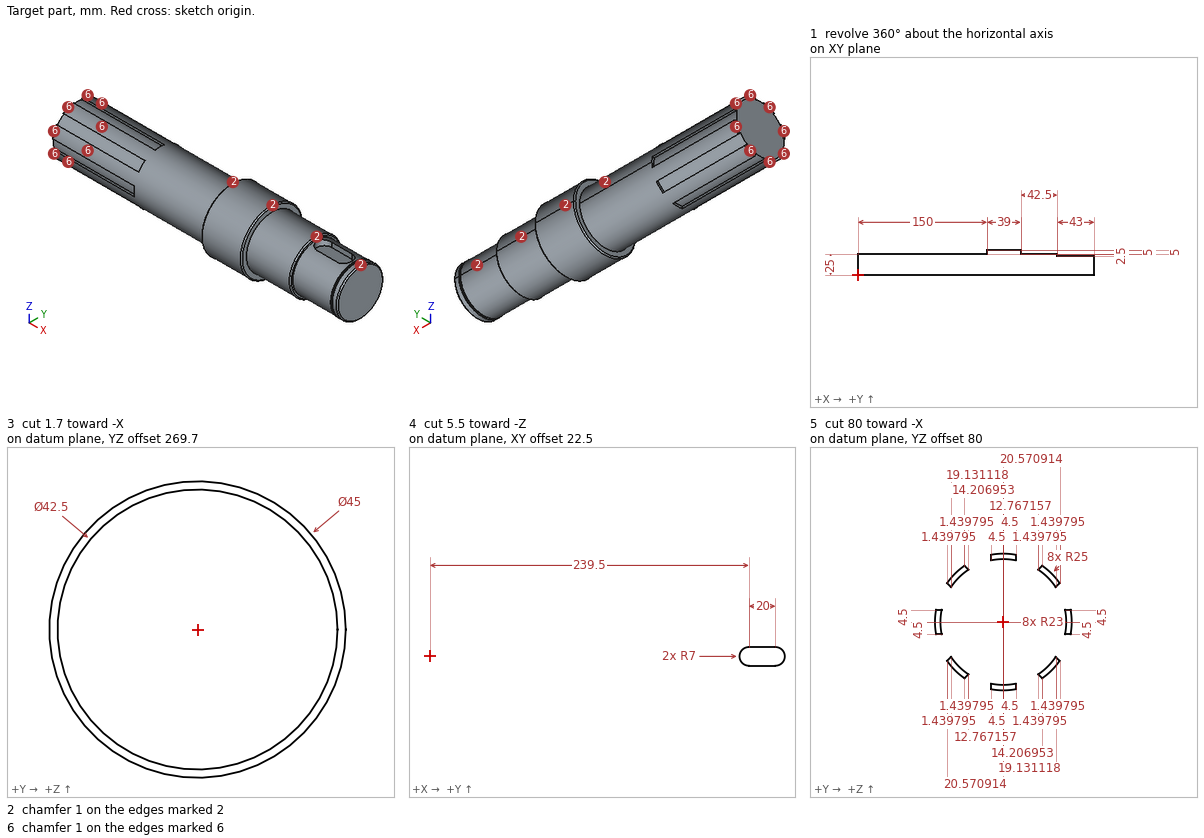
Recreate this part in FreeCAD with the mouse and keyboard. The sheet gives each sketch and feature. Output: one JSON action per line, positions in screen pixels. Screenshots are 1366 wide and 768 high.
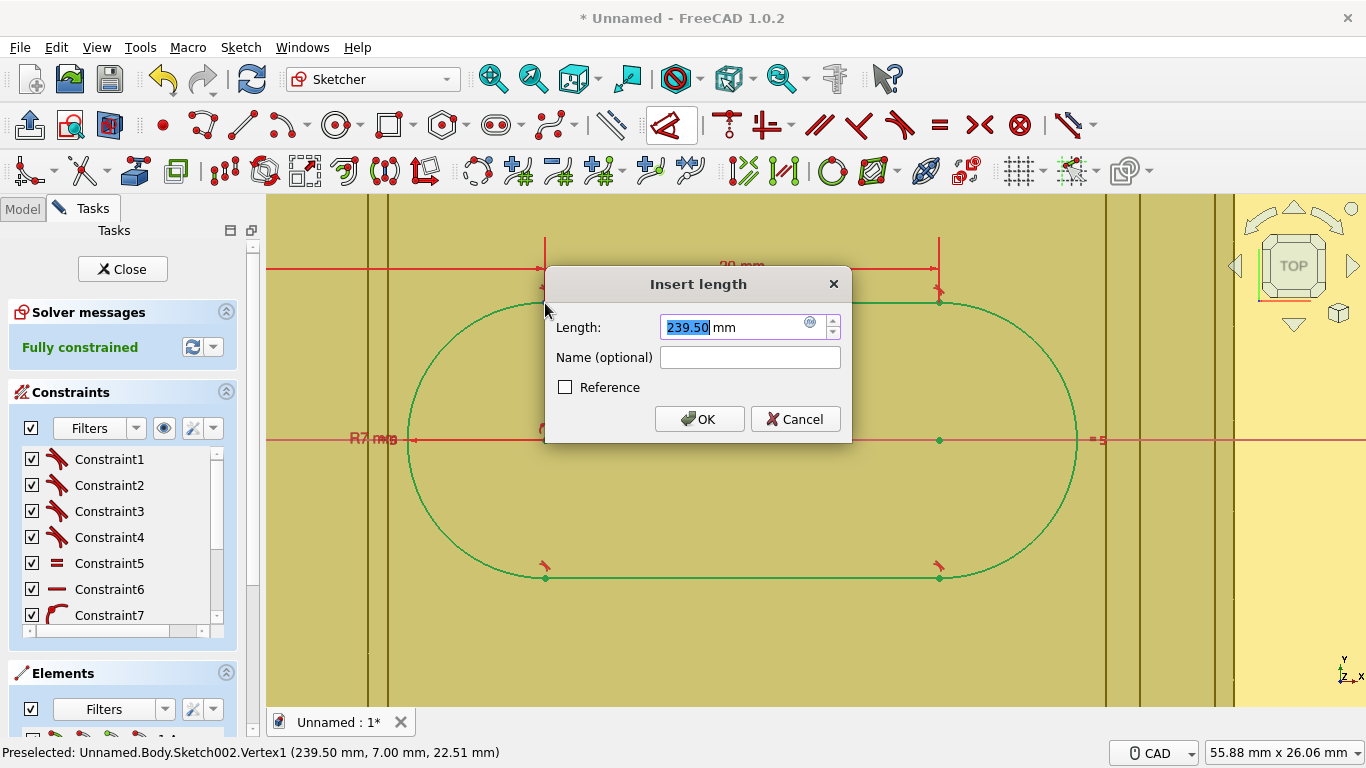
{"action": "type", "text": "239.5"}
{"action": "key", "text": "Return"}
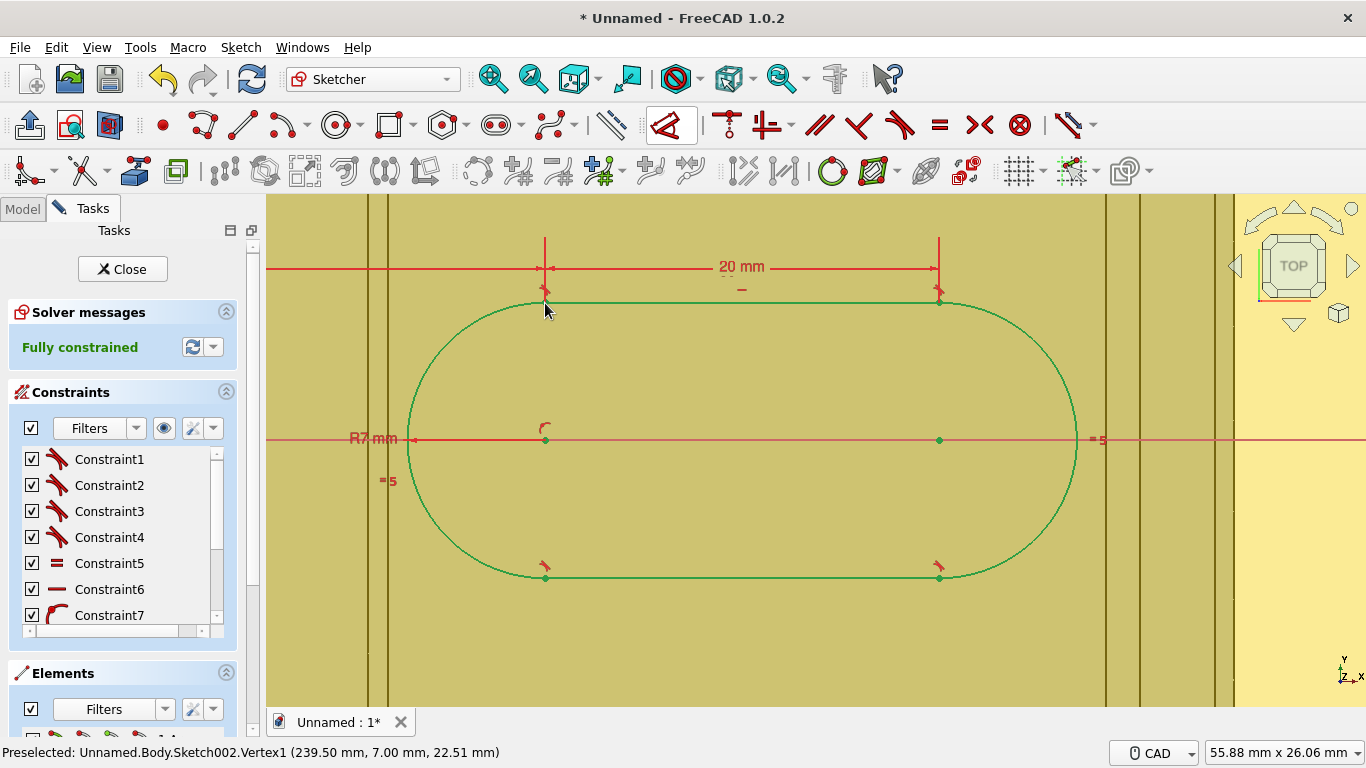
{"action": "left_click", "coordinate": [123, 269]}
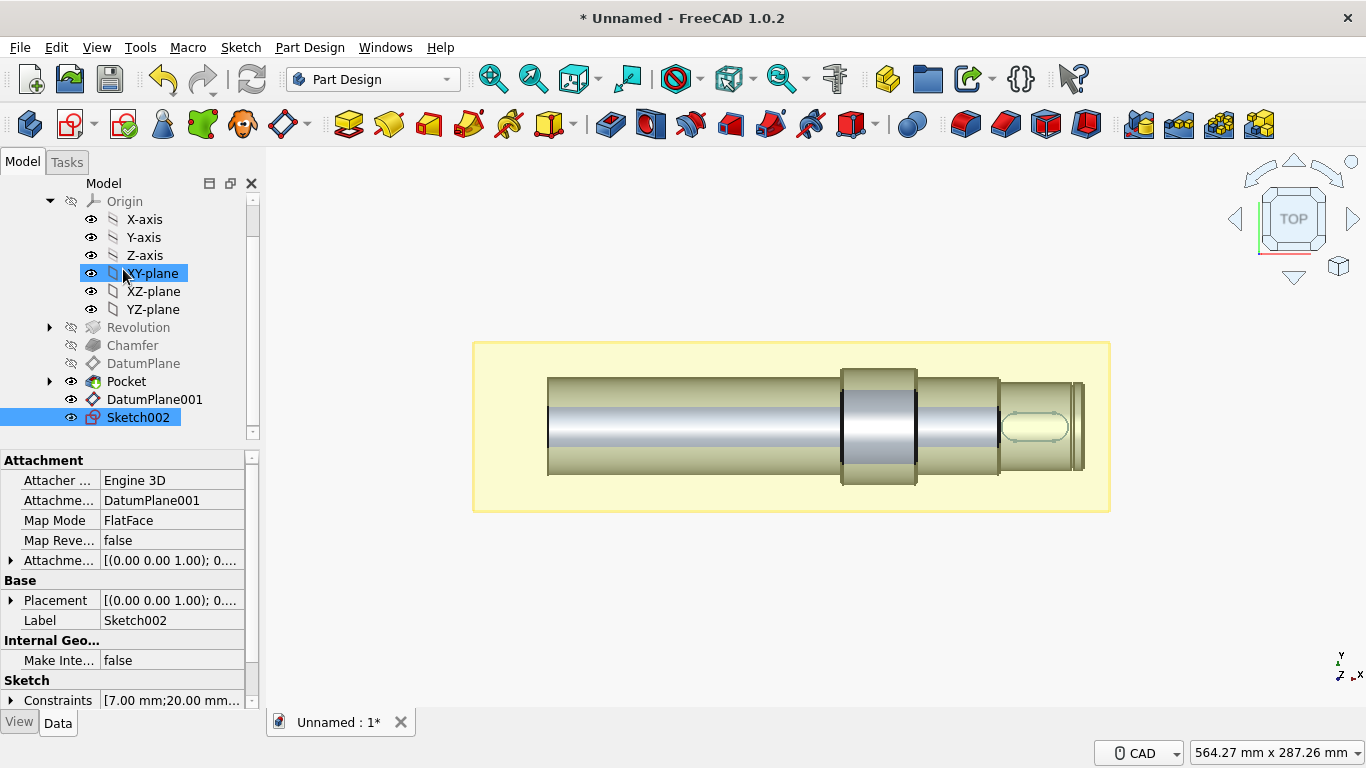
{"action": "left_click", "coordinate": [612, 124]}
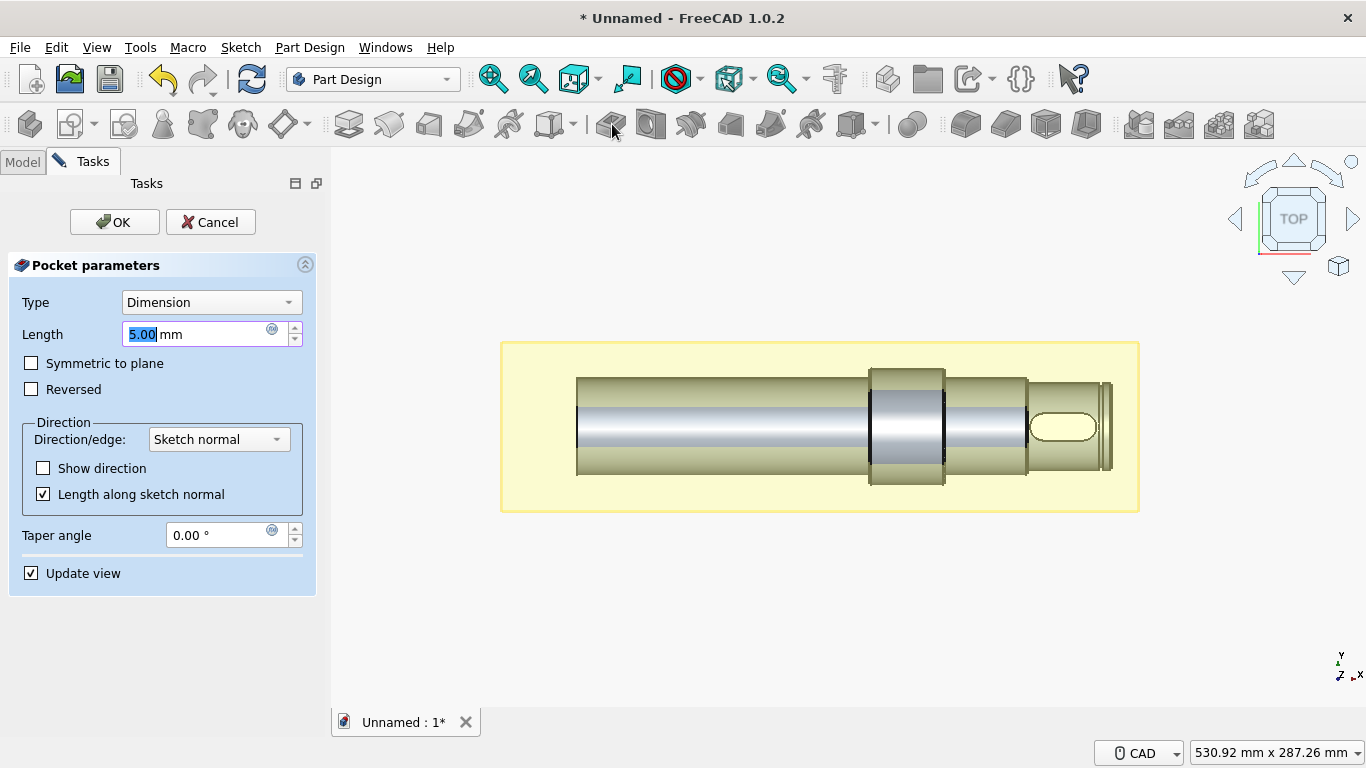
{"action": "type", "text": "5.5"}
{"action": "key", "text": "Tab"}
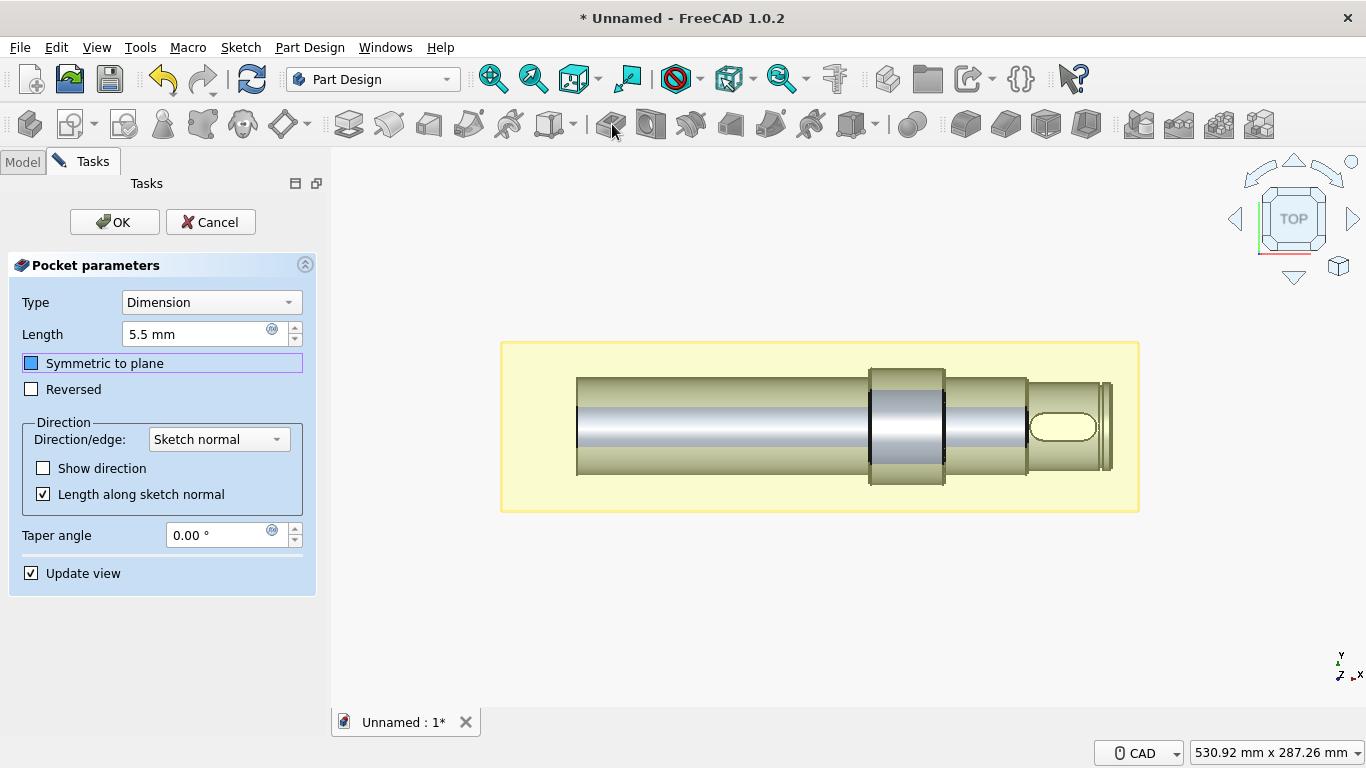
{"action": "left_click", "coordinate": [115, 222]}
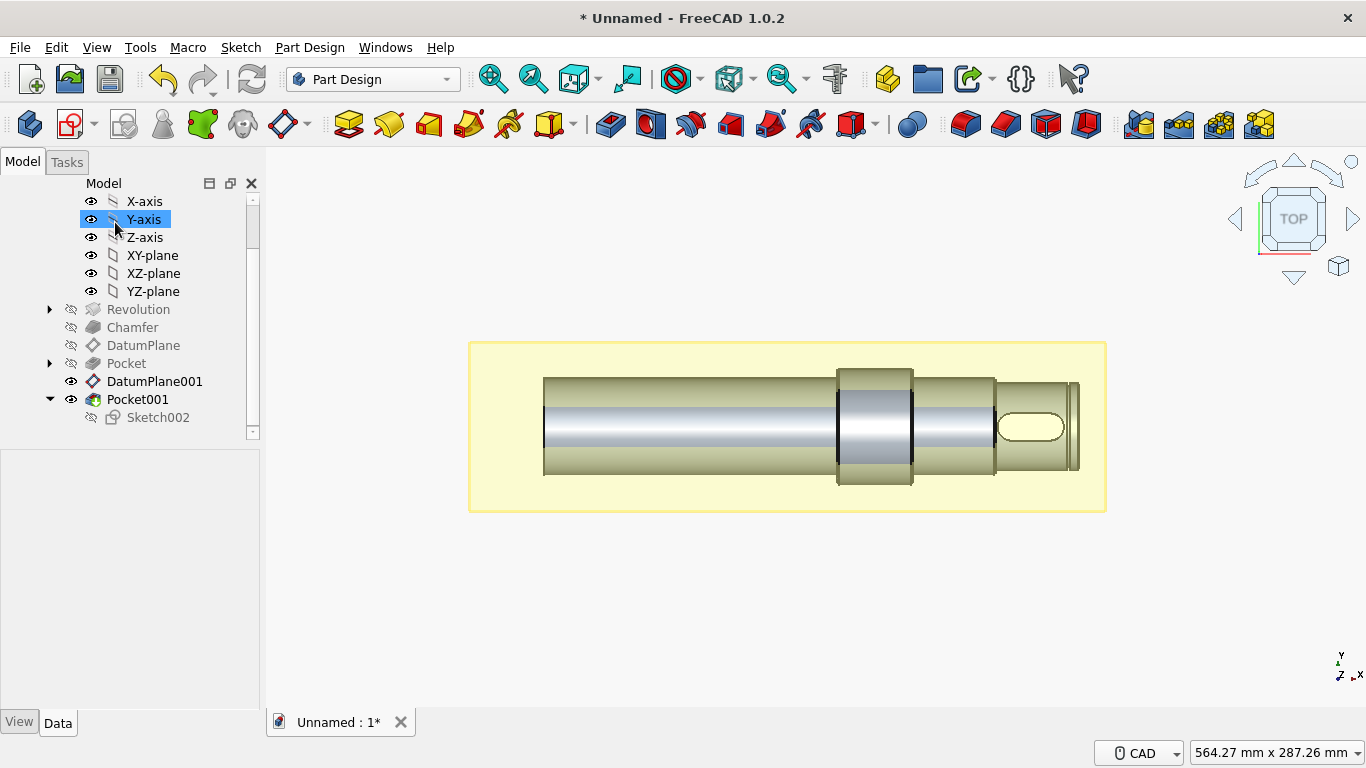
{"action": "left_click", "coordinate": [116, 381]}
{"action": "key", "text": "space"}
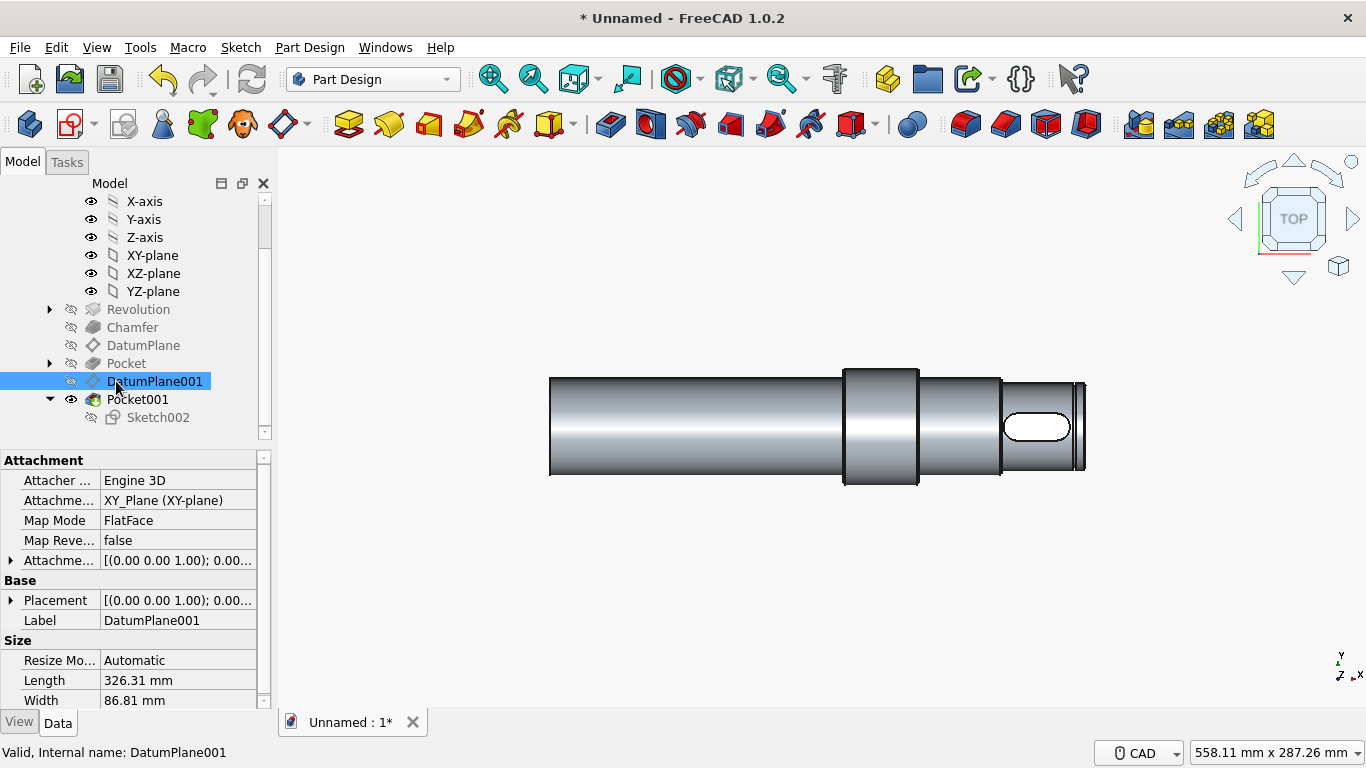
{"action": "scroll", "coordinate": [160, 305], "scroll_direction": "down", "scroll_amount": 3}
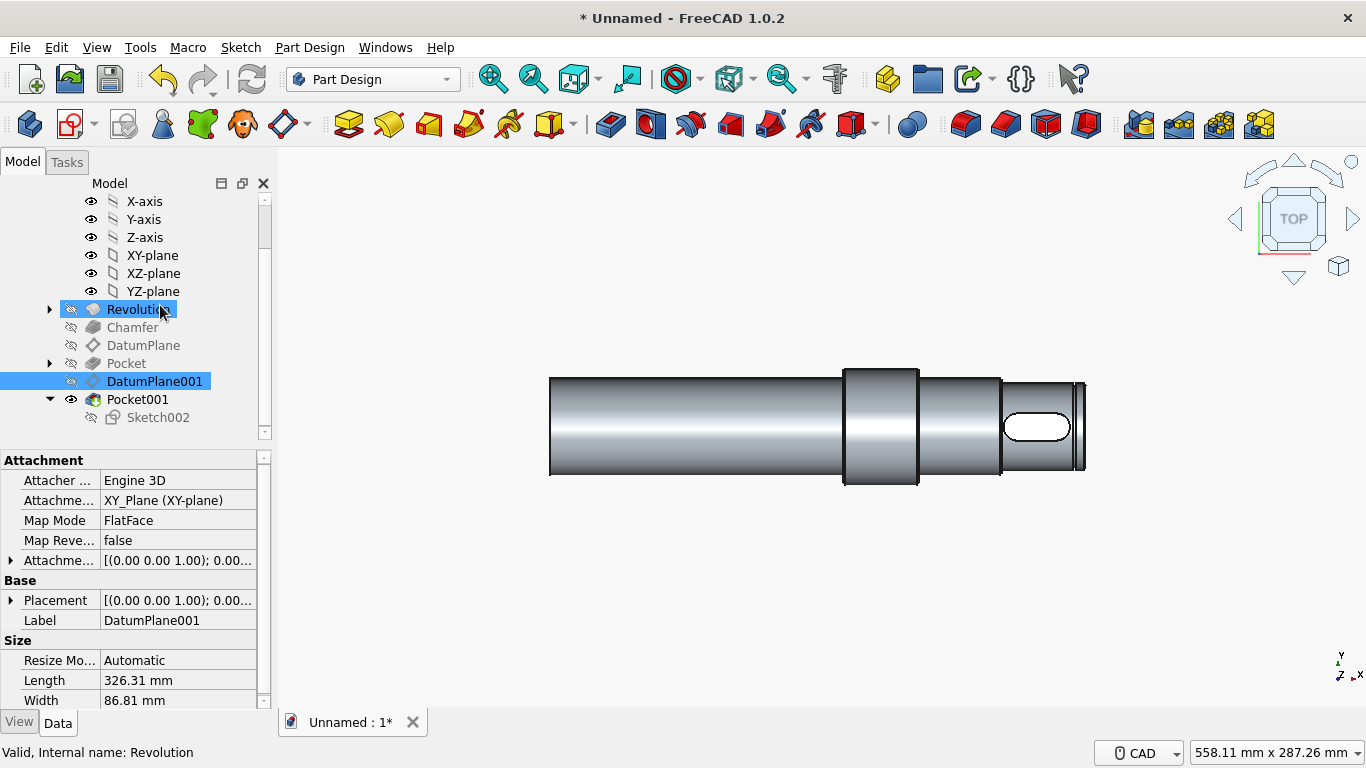
{"action": "scroll", "coordinate": [160, 305], "scroll_direction": "up", "scroll_amount": 15}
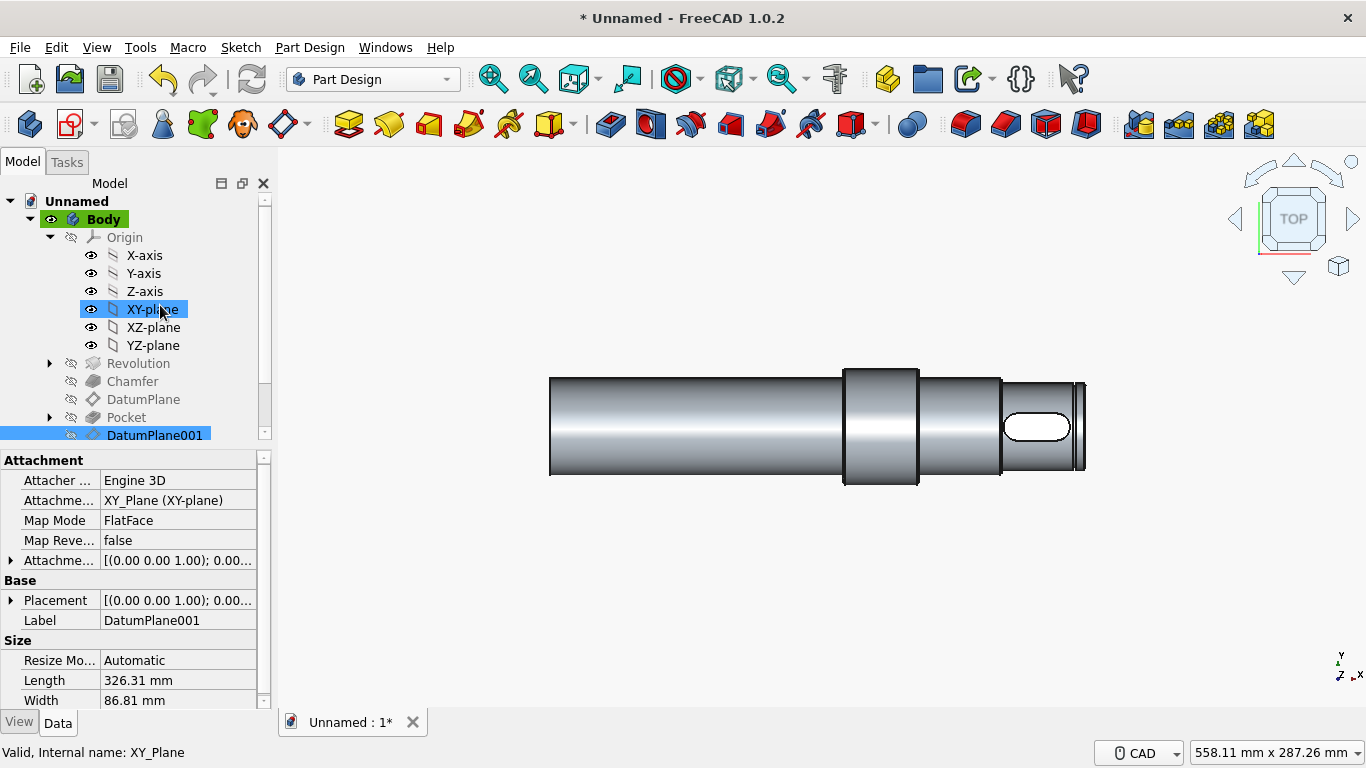
{"action": "left_click", "coordinate": [136, 345]}